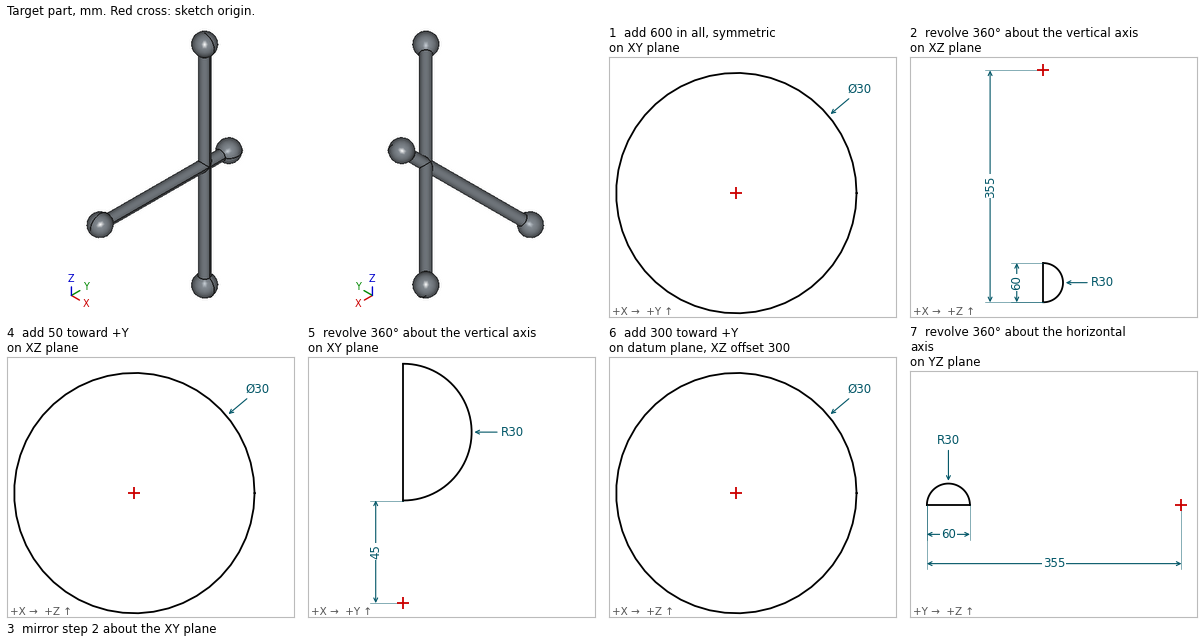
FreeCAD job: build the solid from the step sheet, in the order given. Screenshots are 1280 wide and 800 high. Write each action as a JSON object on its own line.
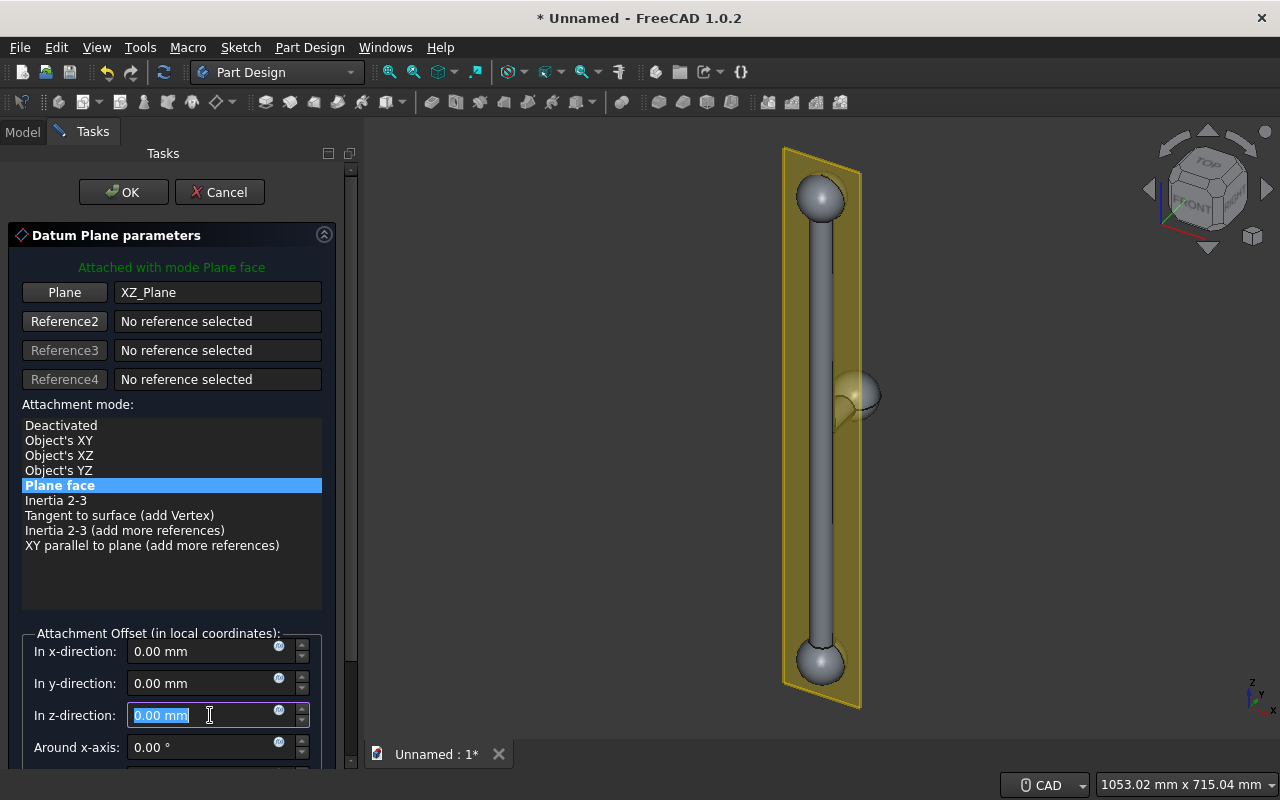
{"action": "type", "text": "300"}
{"action": "key", "text": "Tab"}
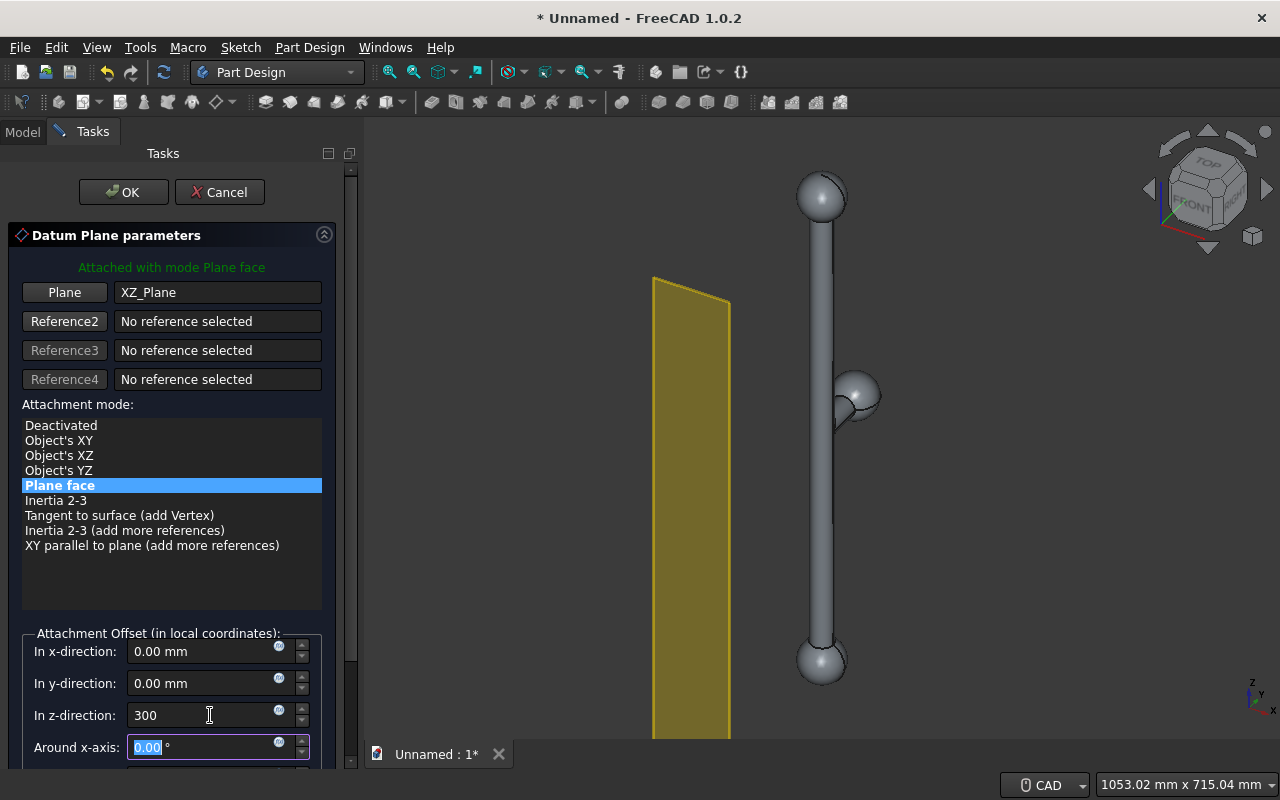
{"action": "left_click", "coordinate": [124, 192]}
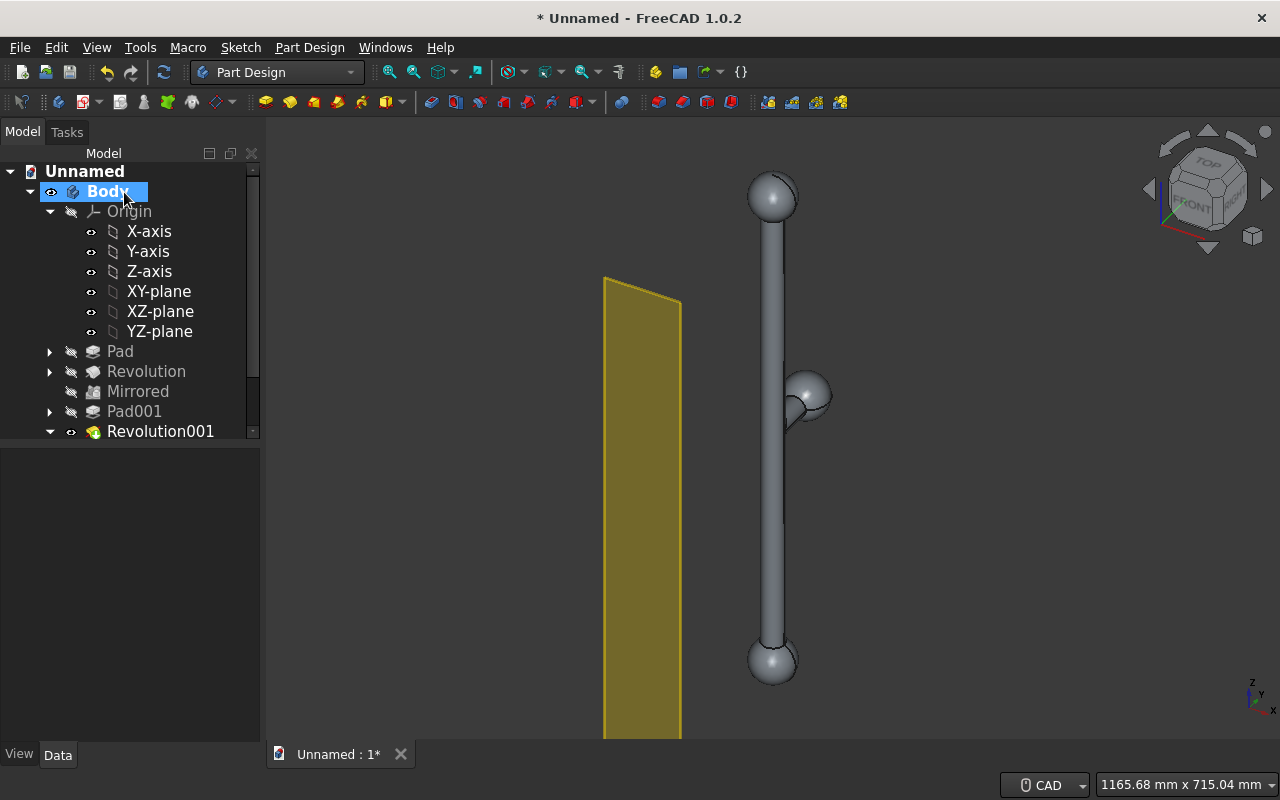
{"action": "scroll", "coordinate": [100, 307], "scroll_direction": "down", "scroll_amount": 3}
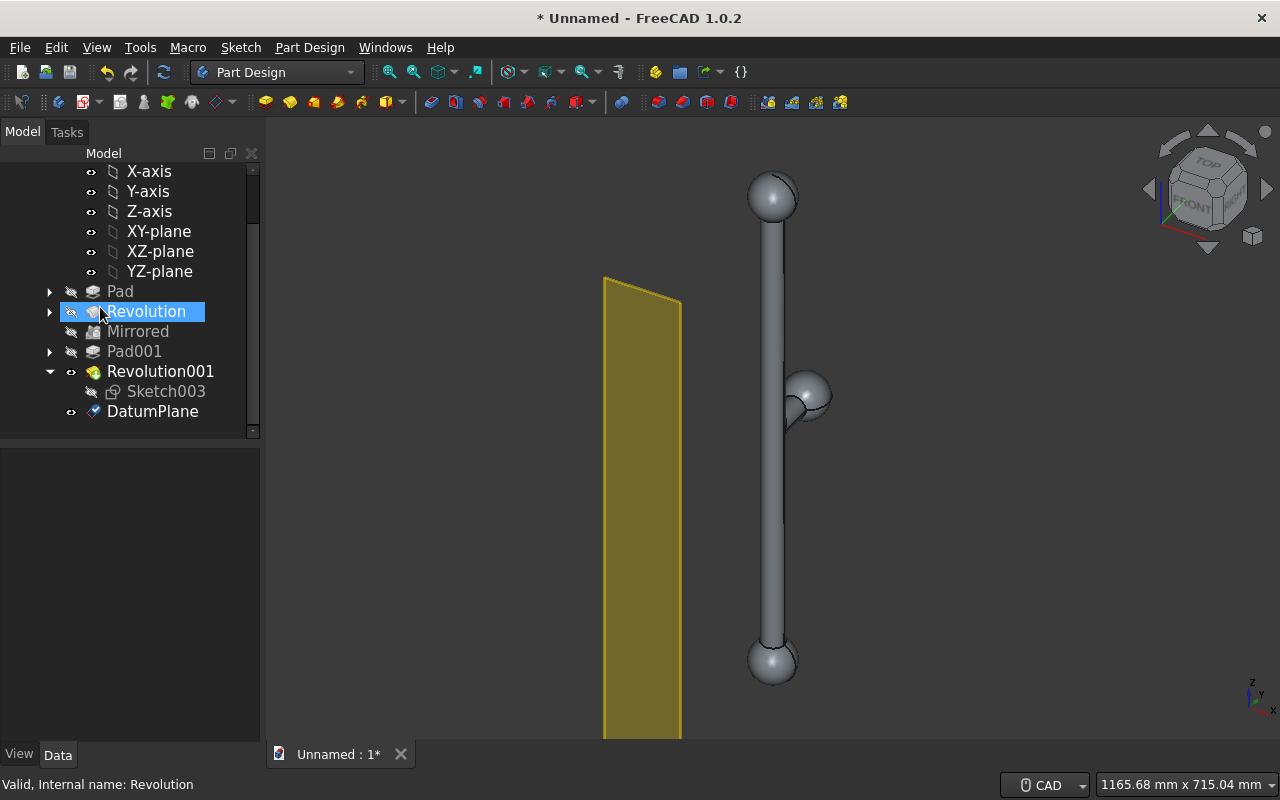
{"action": "left_click", "coordinate": [116, 412]}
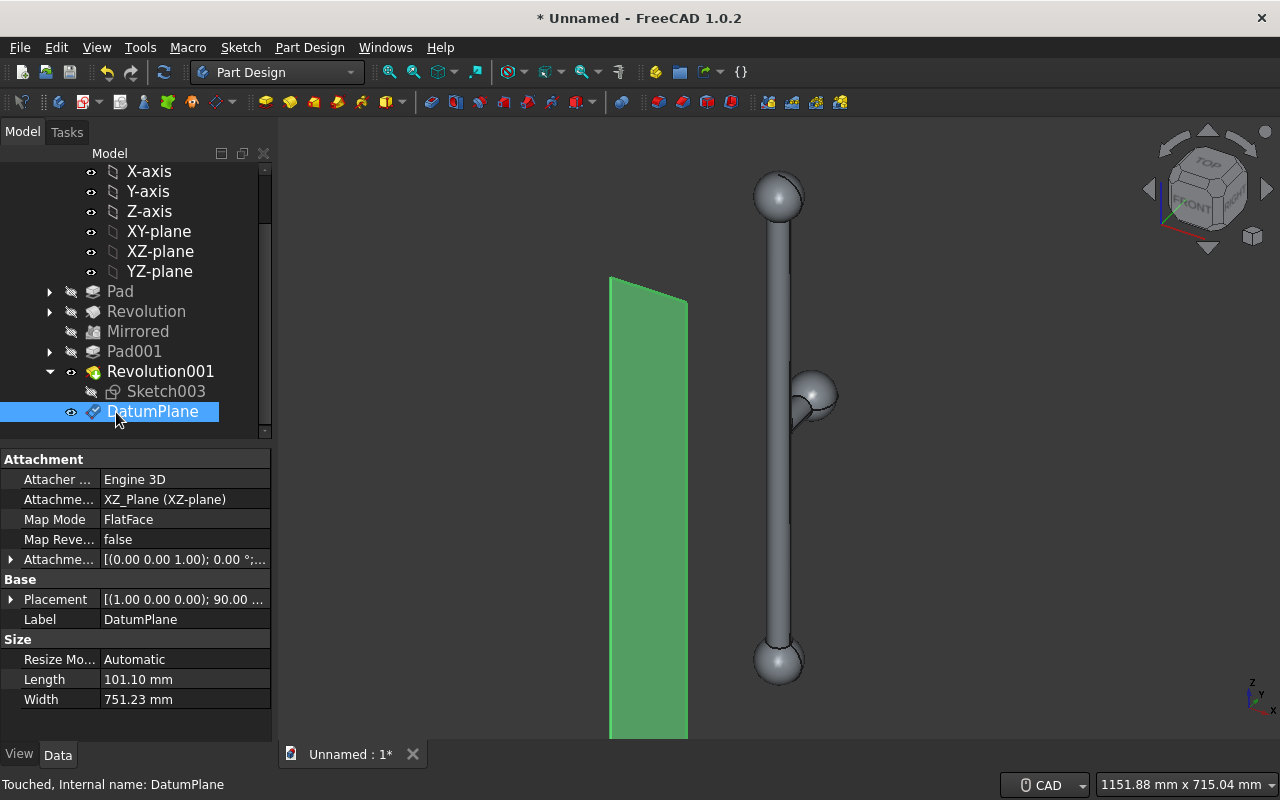
{"action": "left_click", "coordinate": [84, 102]}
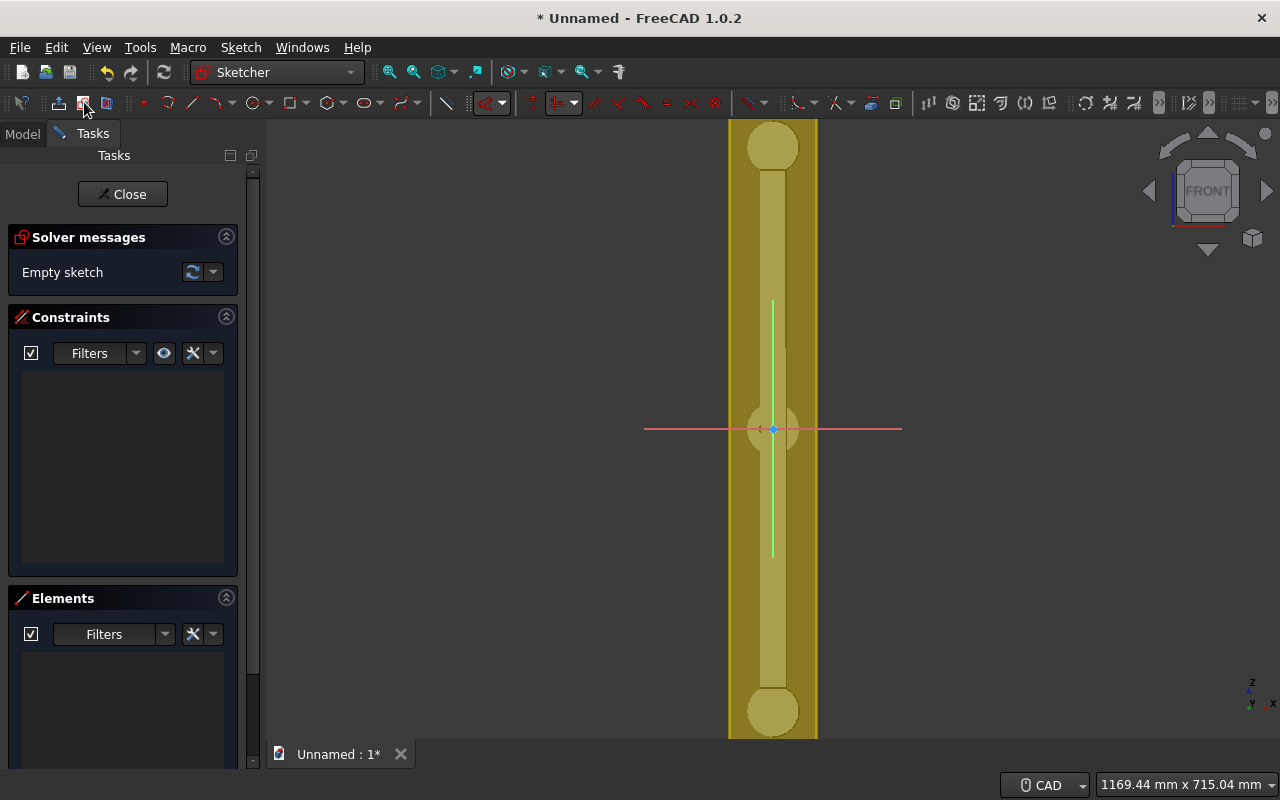
{"action": "scroll", "coordinate": [778, 429], "scroll_direction": "up", "scroll_amount": 14}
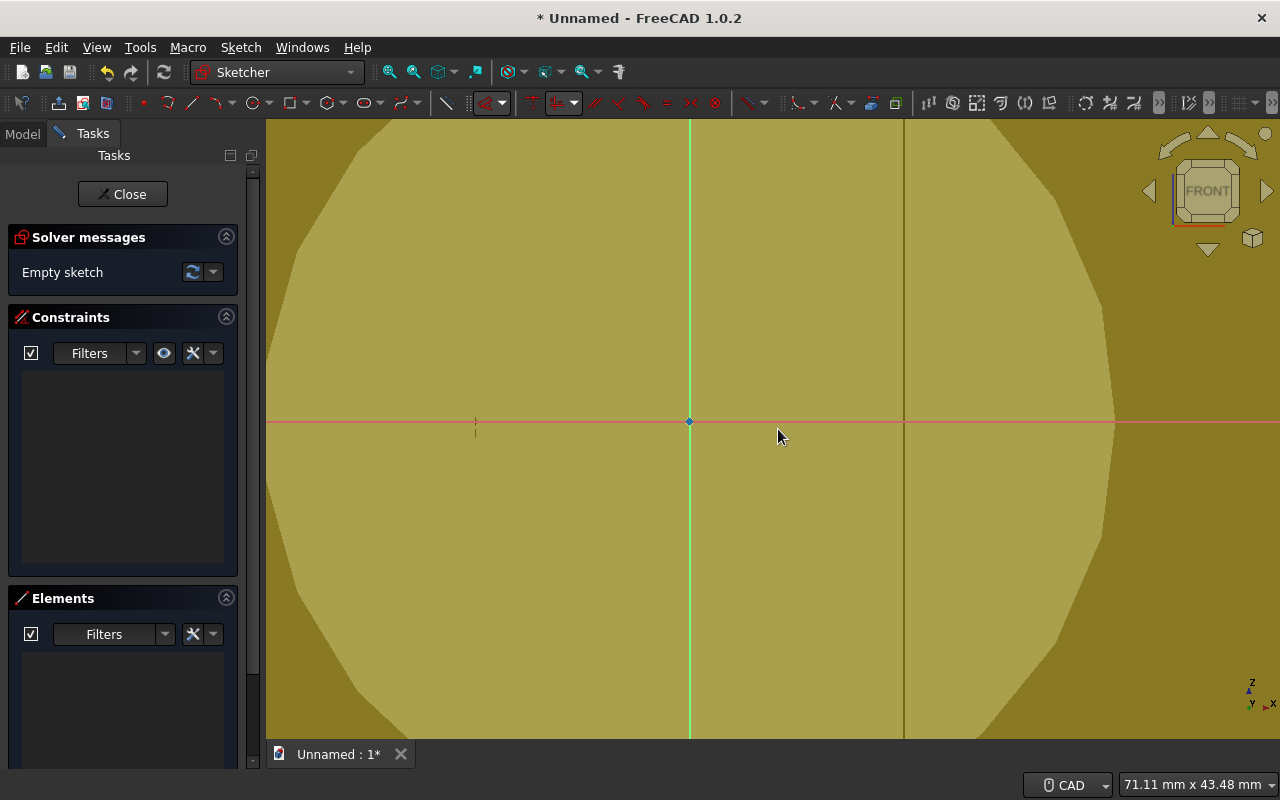
{"action": "left_click", "coordinate": [254, 104]}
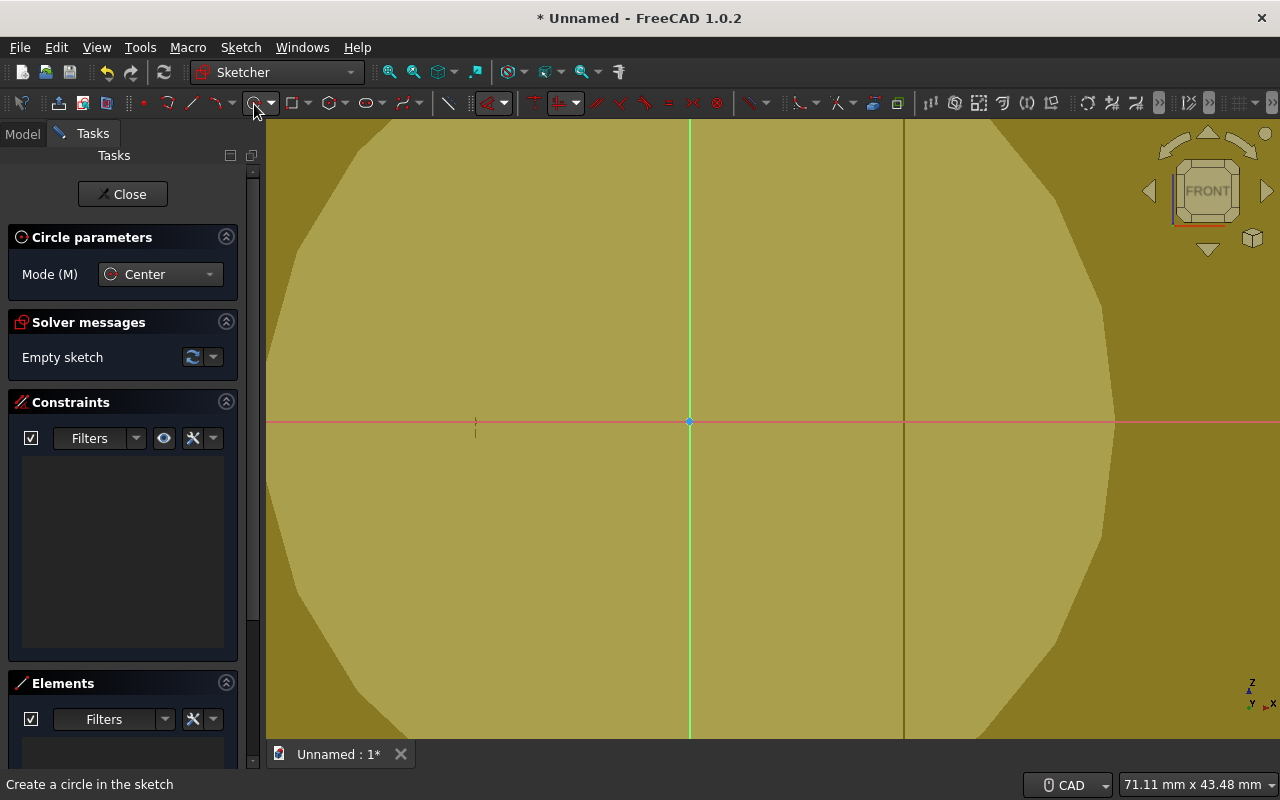
{"action": "left_click", "coordinate": [690, 422]}
{"action": "left_click", "coordinate": [841, 271]}
{"action": "key", "text": "Escape"}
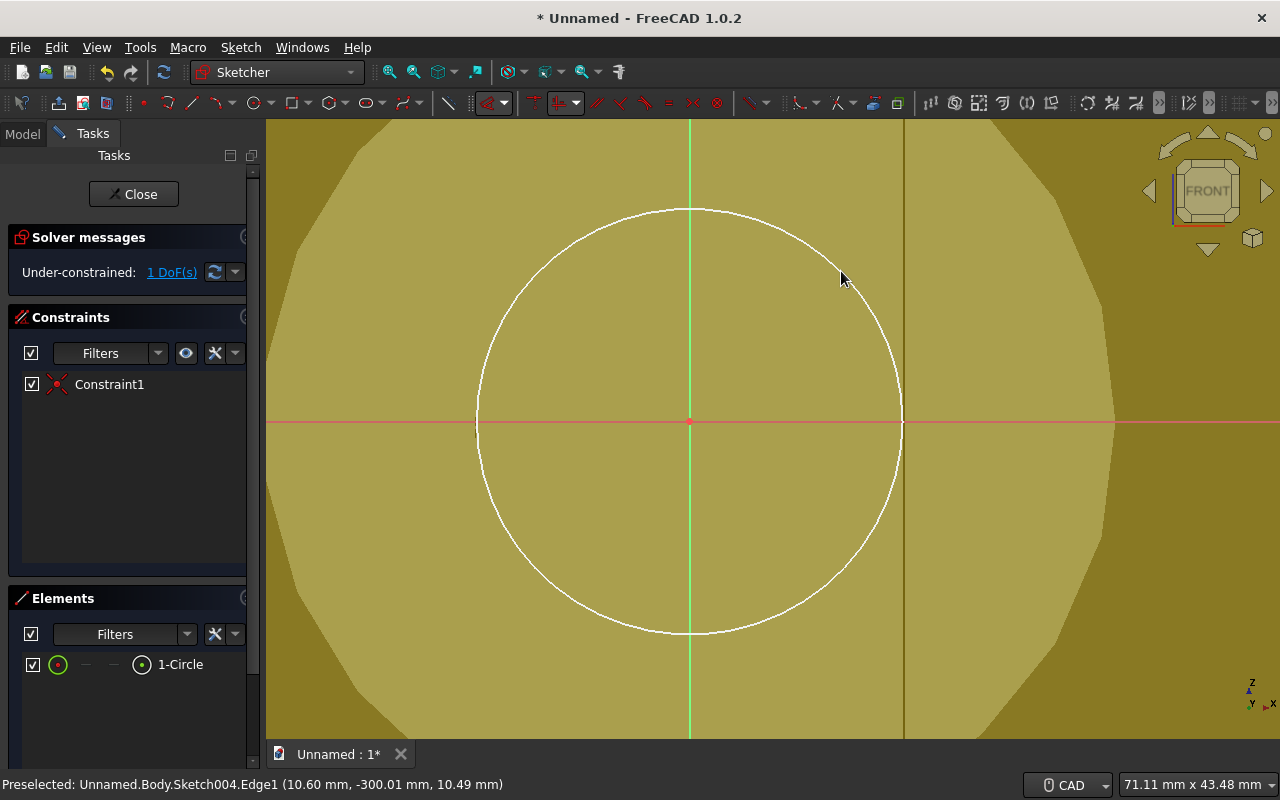
{"action": "left_click", "coordinate": [840, 271]}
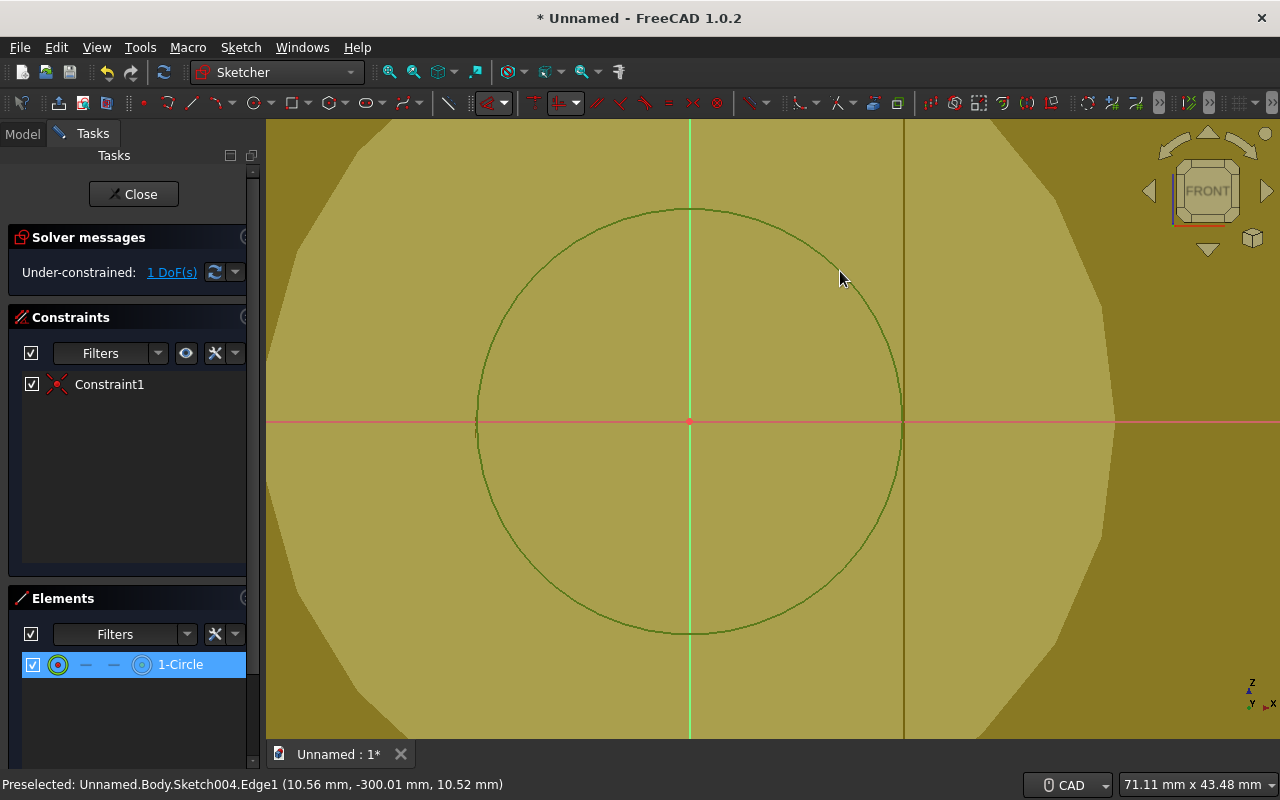
{"action": "left_click", "coordinate": [506, 104]}